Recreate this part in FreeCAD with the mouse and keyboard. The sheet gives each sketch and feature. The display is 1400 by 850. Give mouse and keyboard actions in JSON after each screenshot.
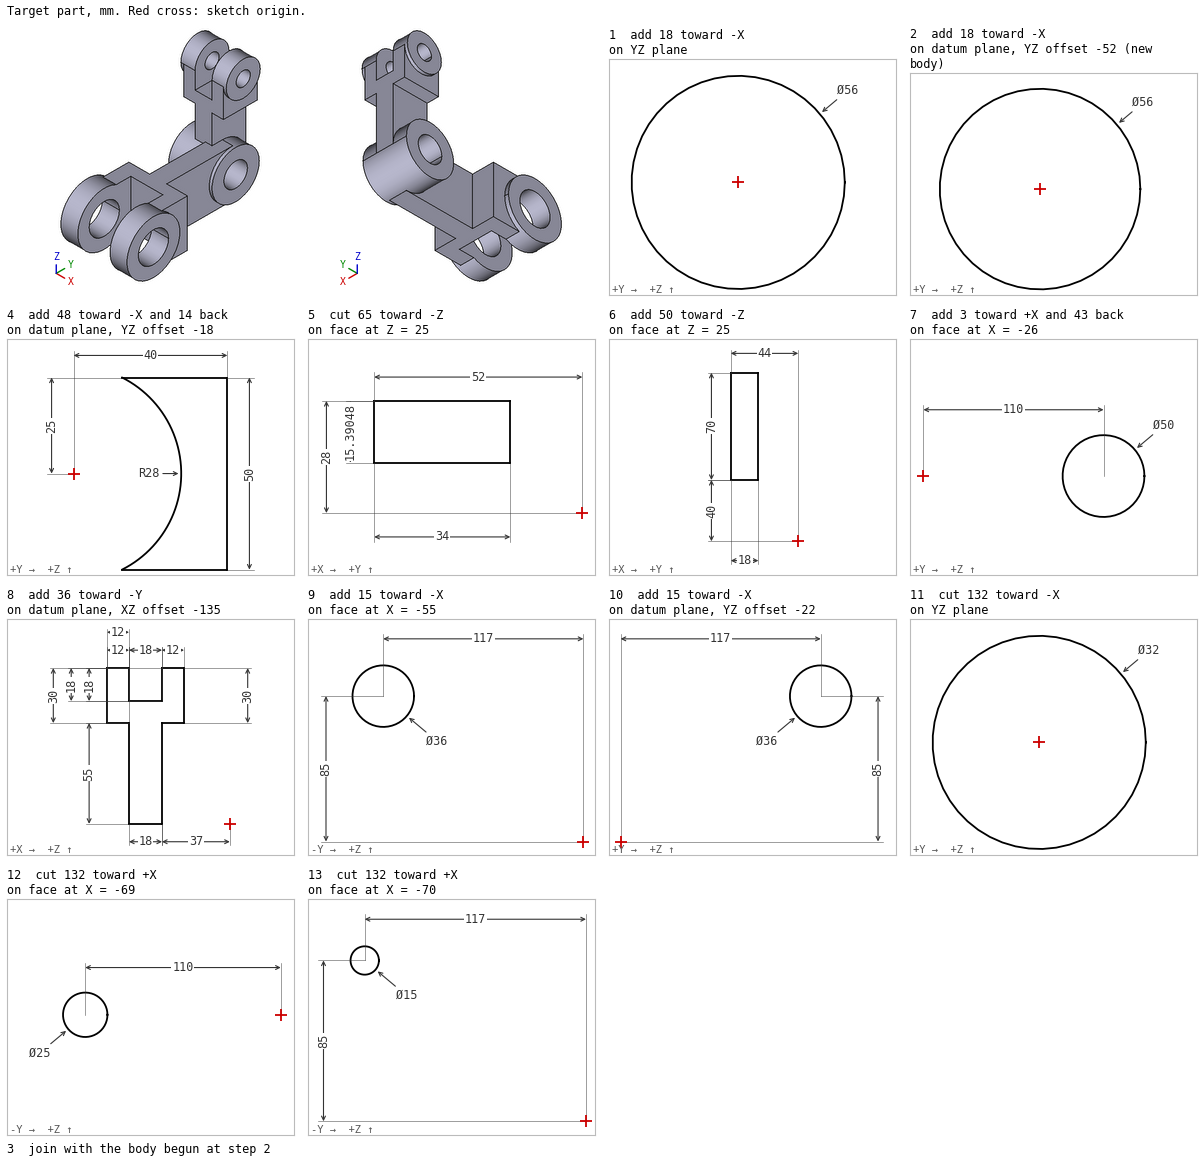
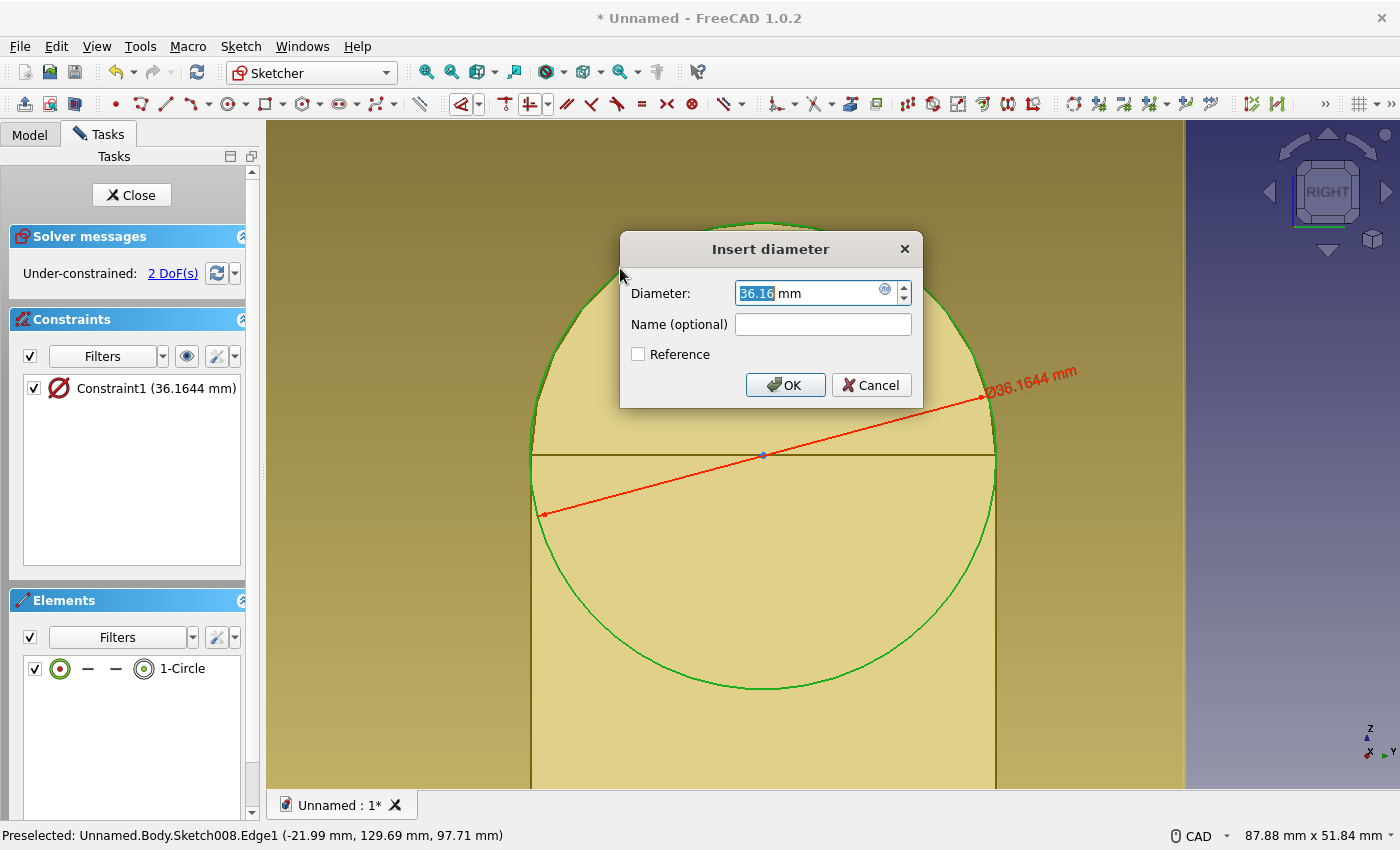
{"action": "type", "text": "36"}
{"action": "key", "text": "Return"}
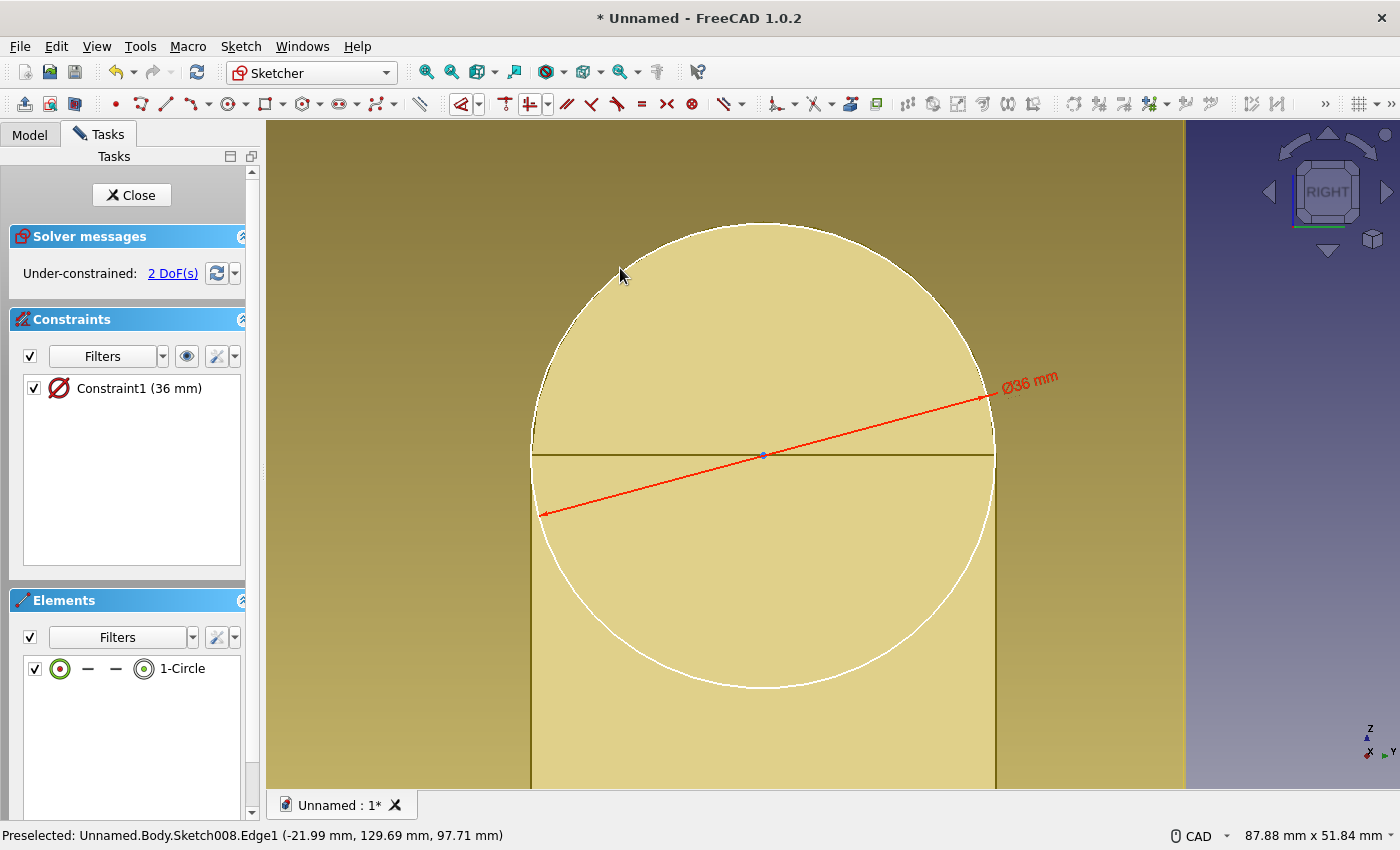
{"action": "left_click", "coordinate": [763, 456]}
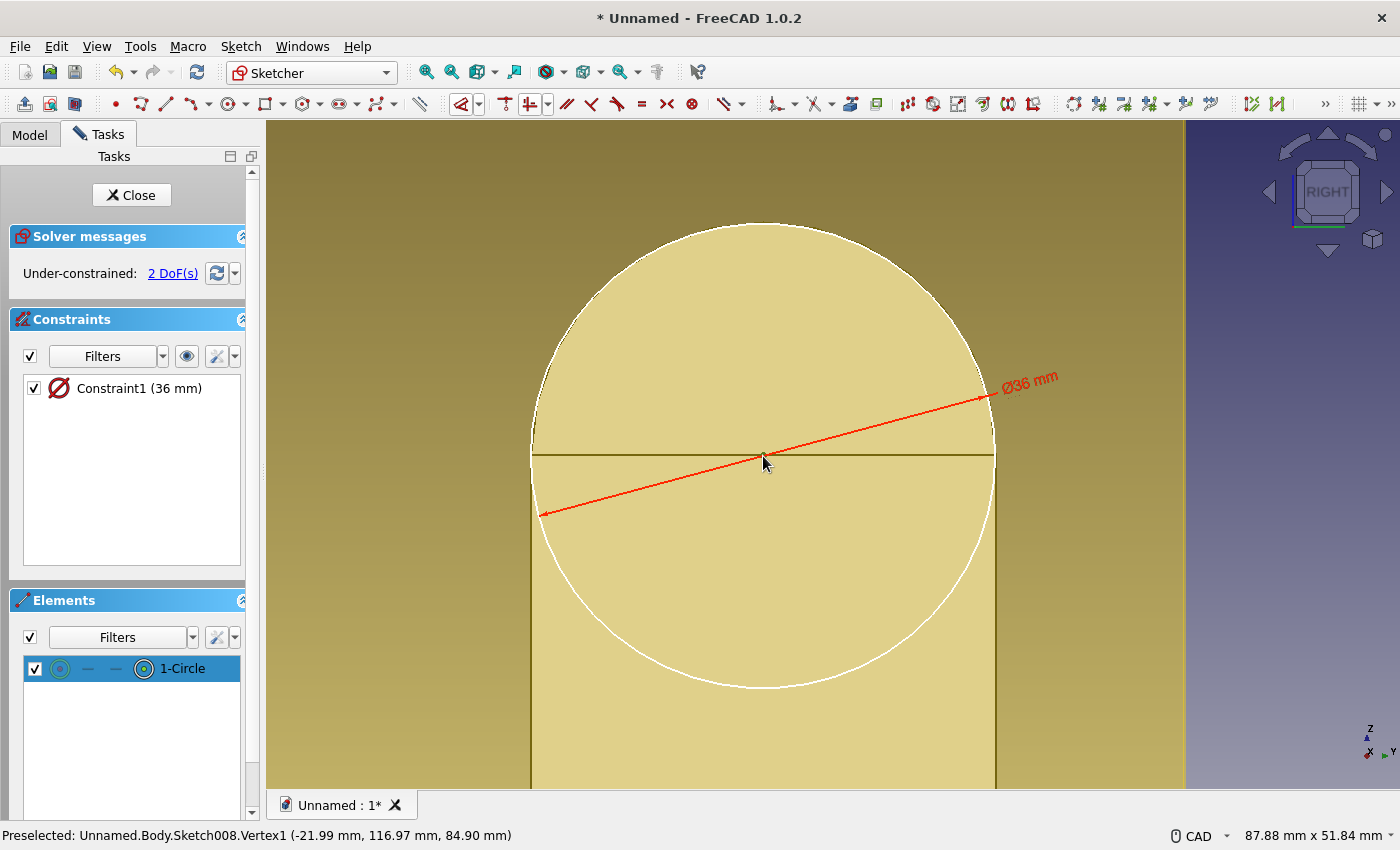
{"action": "key", "text": "i"}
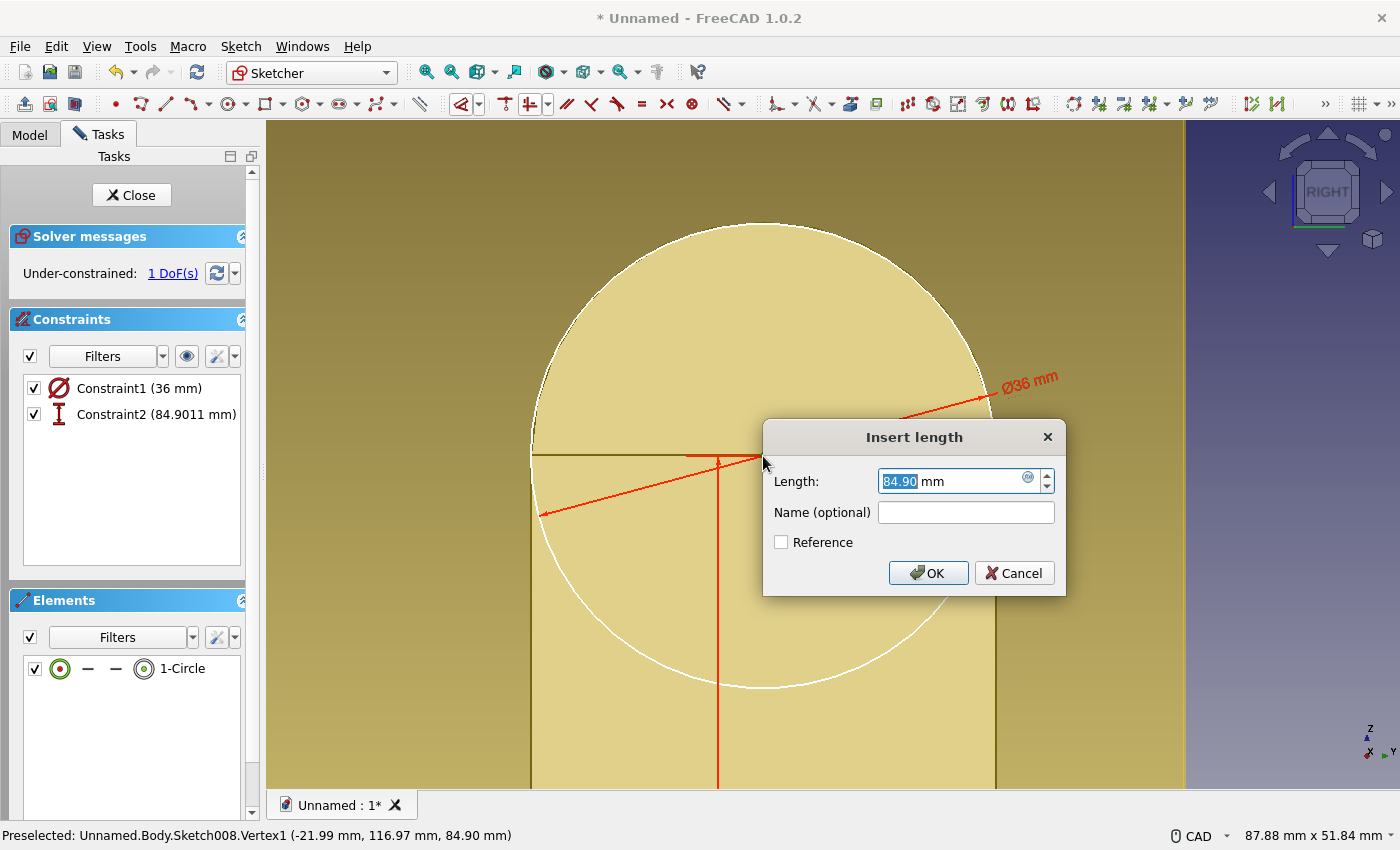
{"action": "type", "text": "85"}
{"action": "key", "text": "Return"}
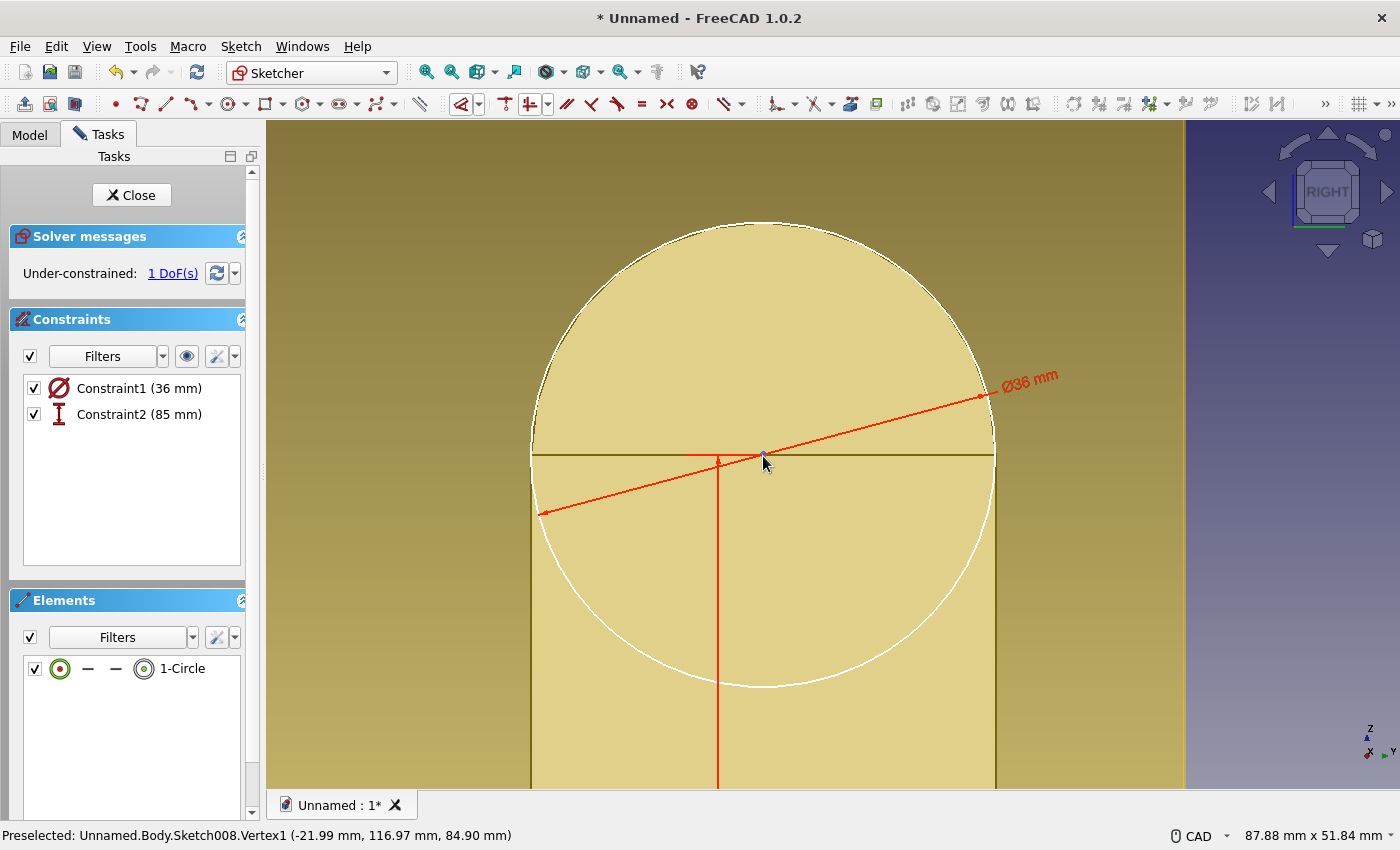
{"action": "left_click", "coordinate": [763, 455]}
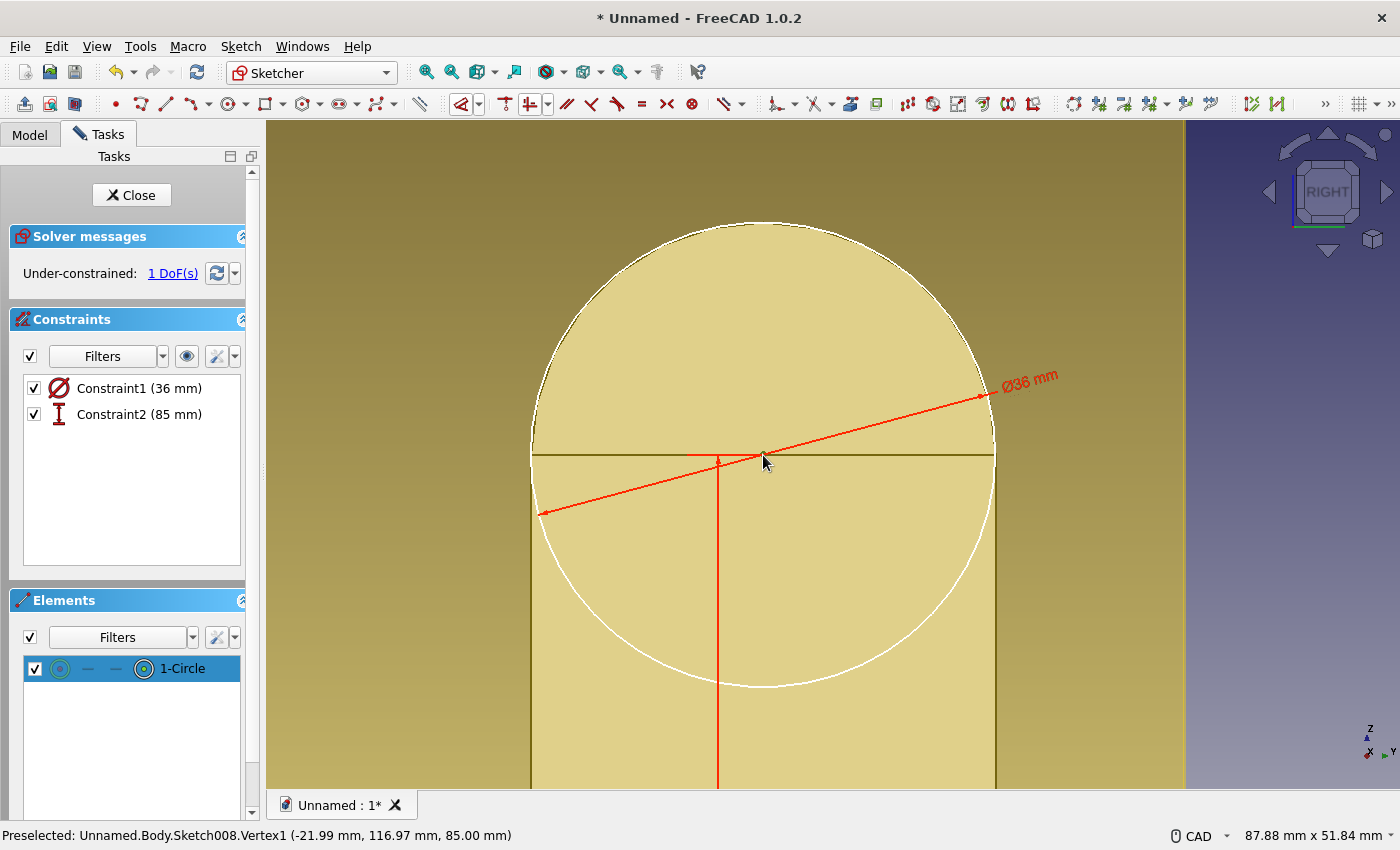
{"action": "key", "text": "l"}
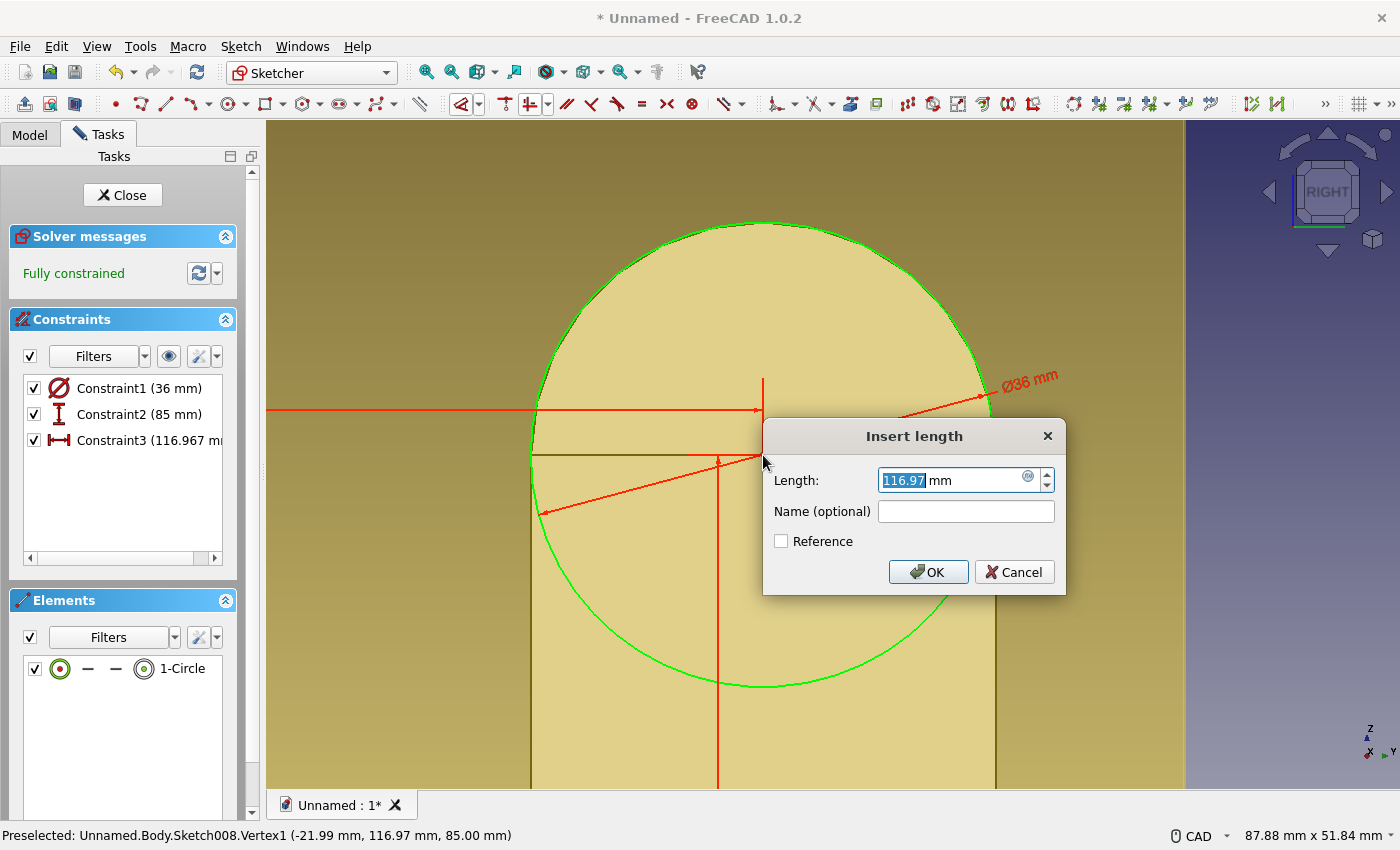
{"action": "type", "text": "117"}
{"action": "key", "text": "Return"}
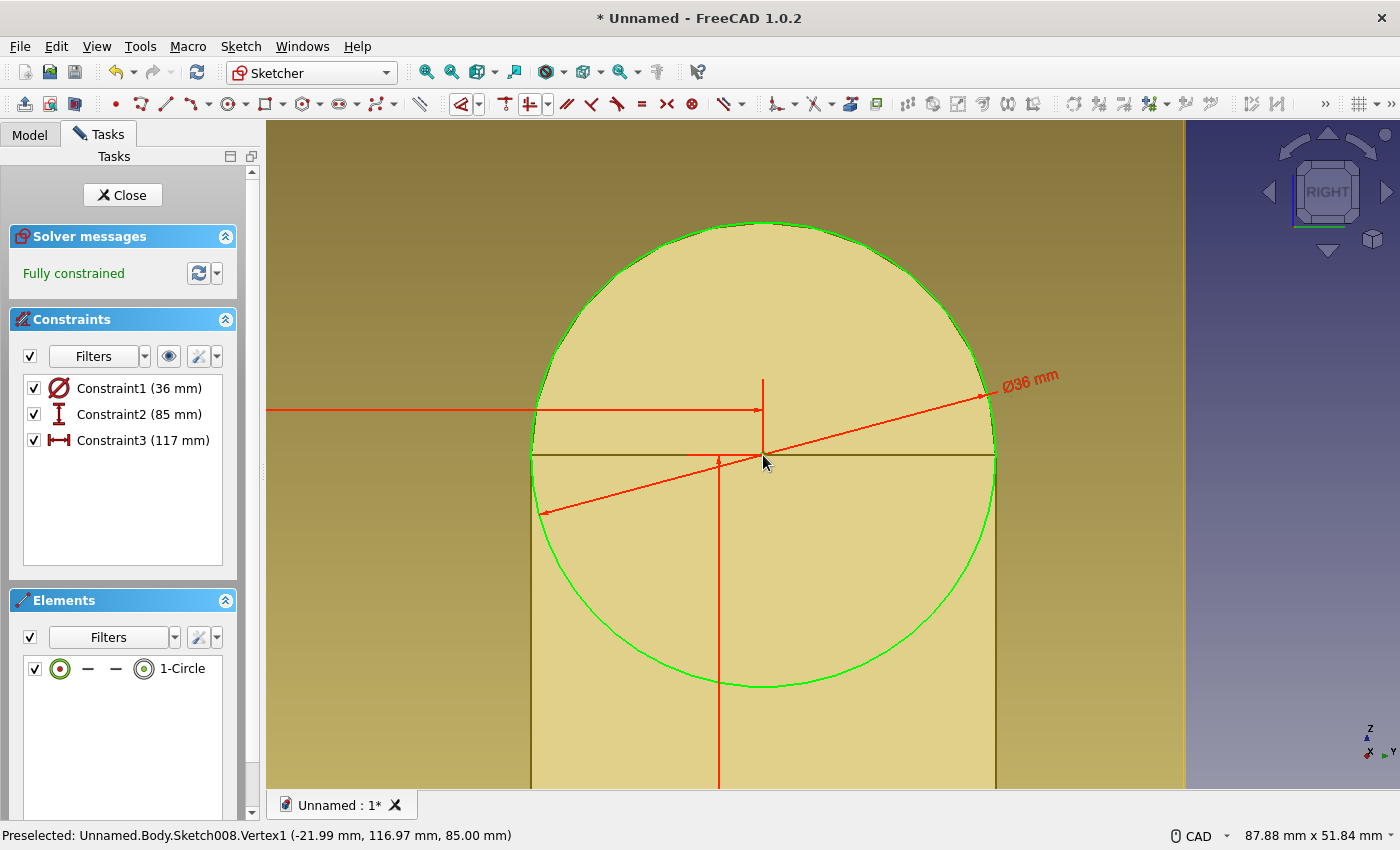
{"action": "left_click", "coordinate": [123, 195]}